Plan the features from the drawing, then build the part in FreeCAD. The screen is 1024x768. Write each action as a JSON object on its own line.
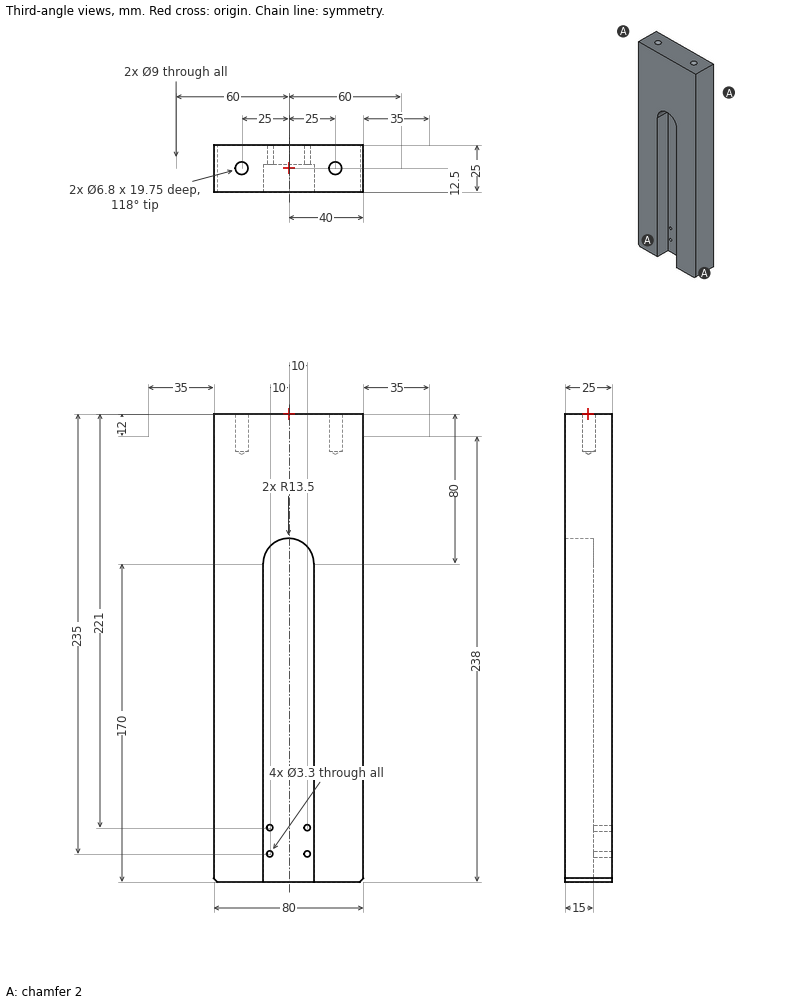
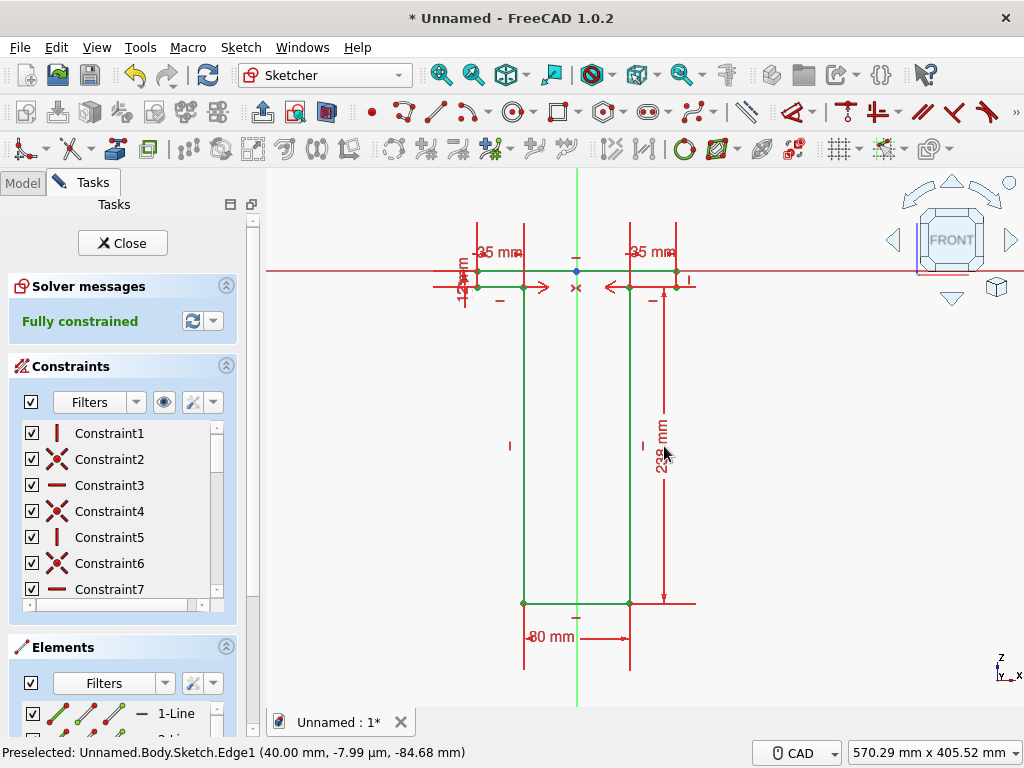
{"action": "left_click", "coordinate": [123, 243]}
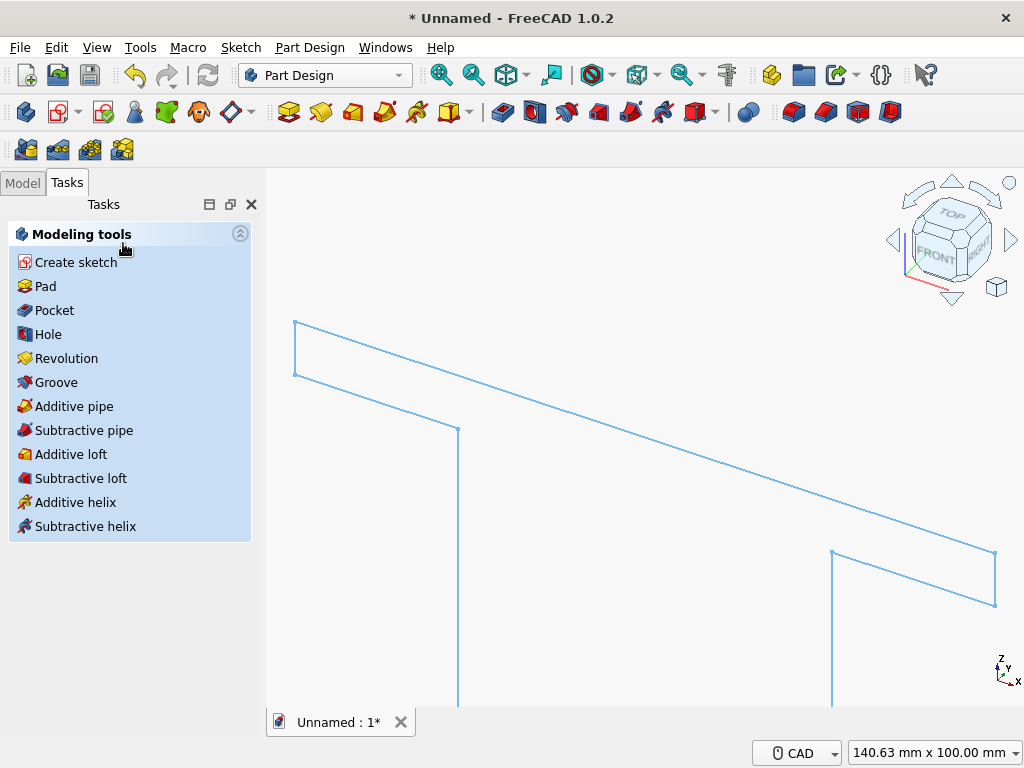
{"action": "left_click", "coordinate": [290, 112]}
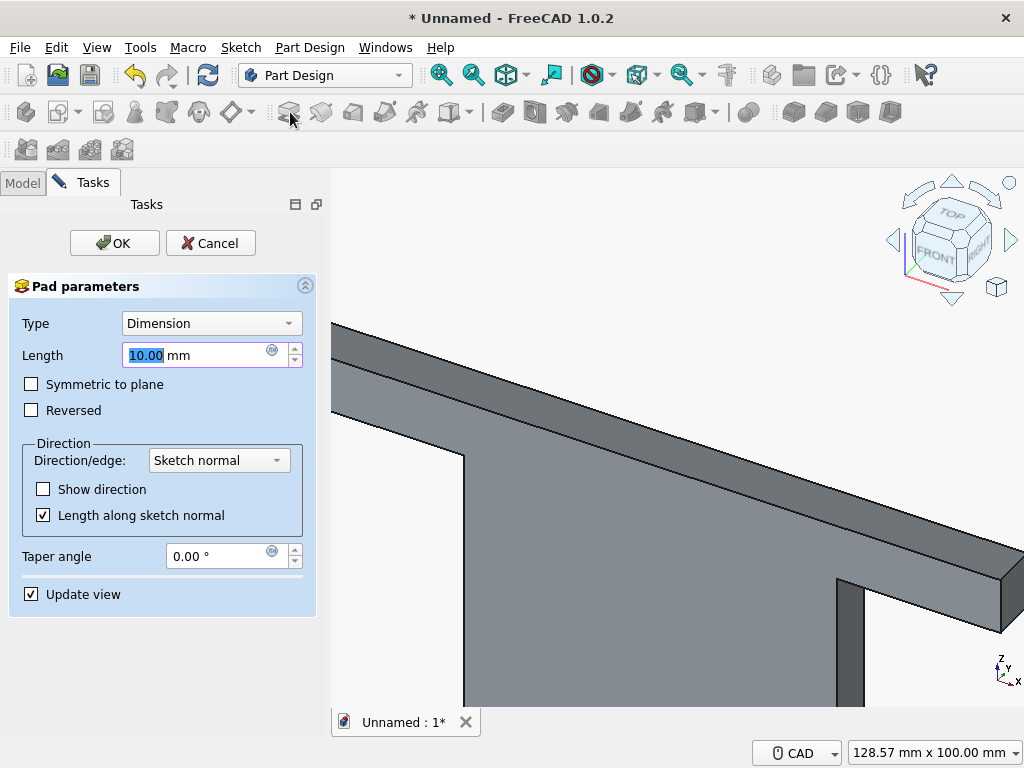
{"action": "type", "text": "25"}
{"action": "key", "text": "Tab"}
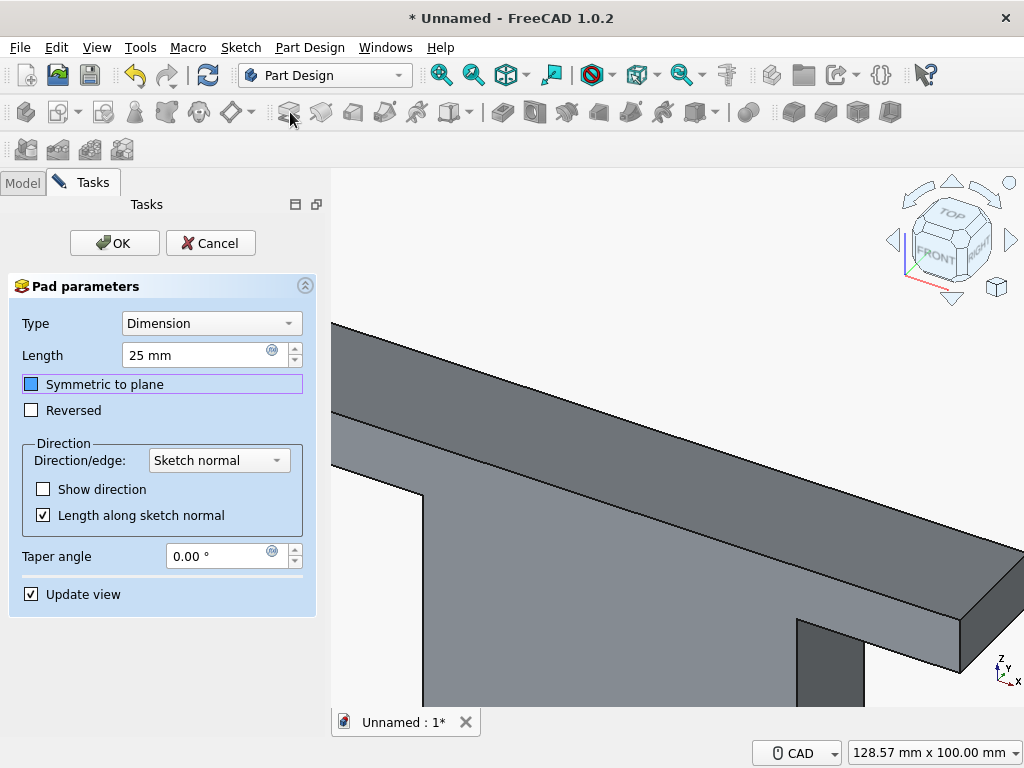
{"action": "left_click", "coordinate": [30, 384]}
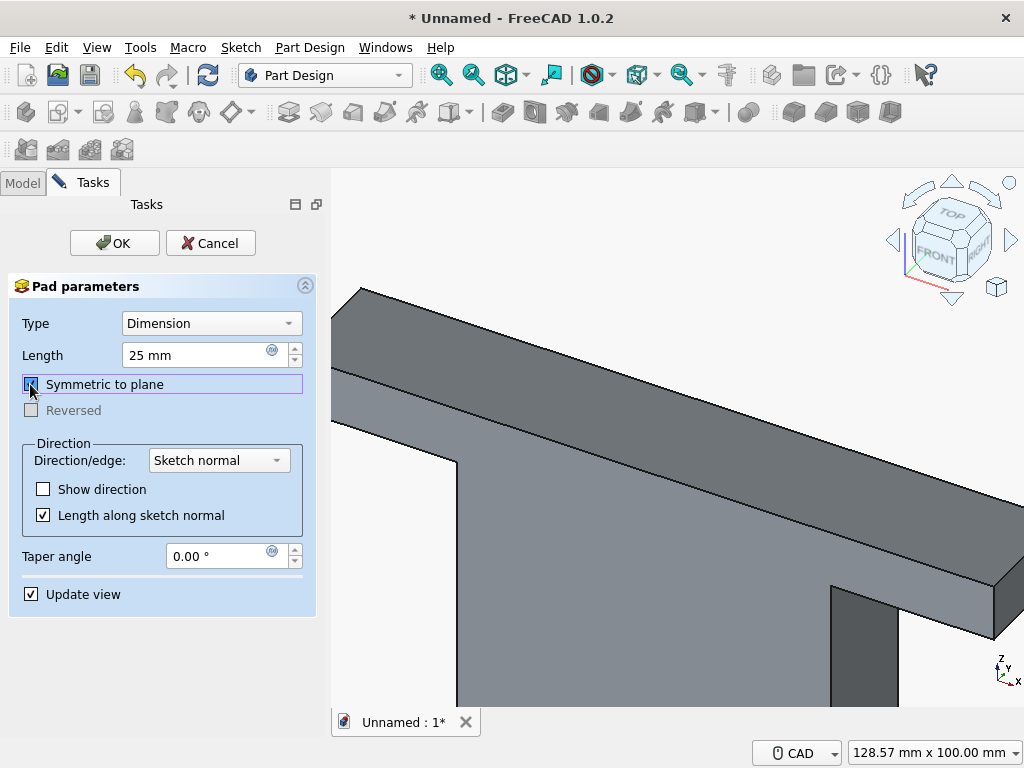
{"action": "left_click", "coordinate": [115, 243]}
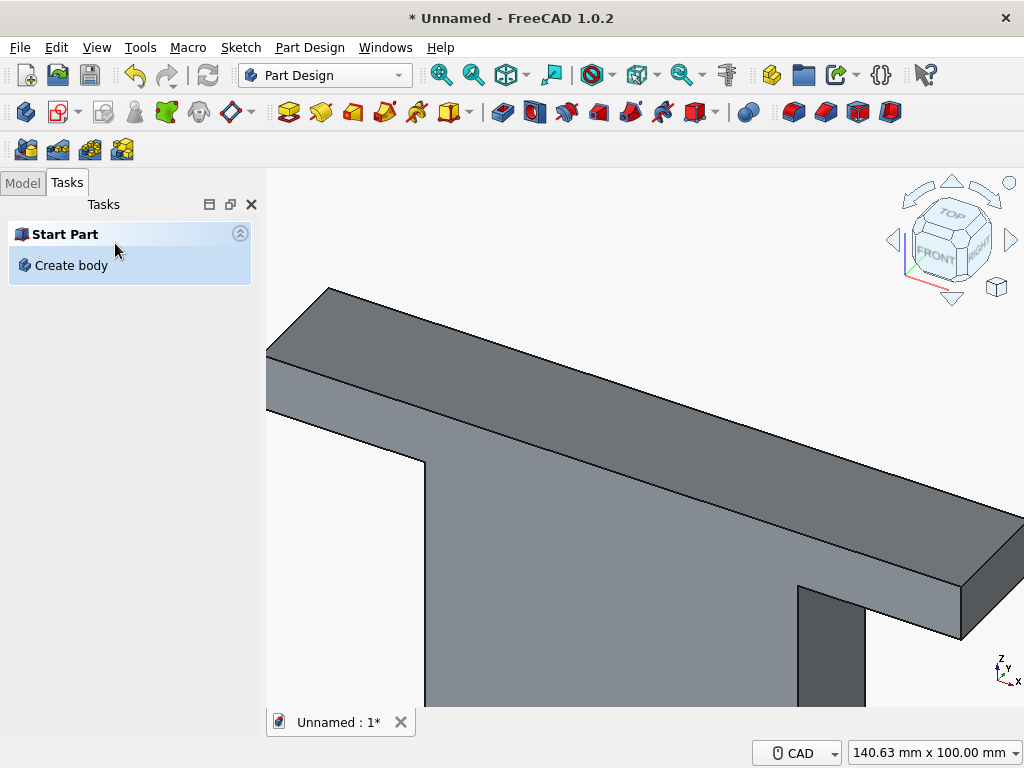
{"action": "key", "text": "v f"}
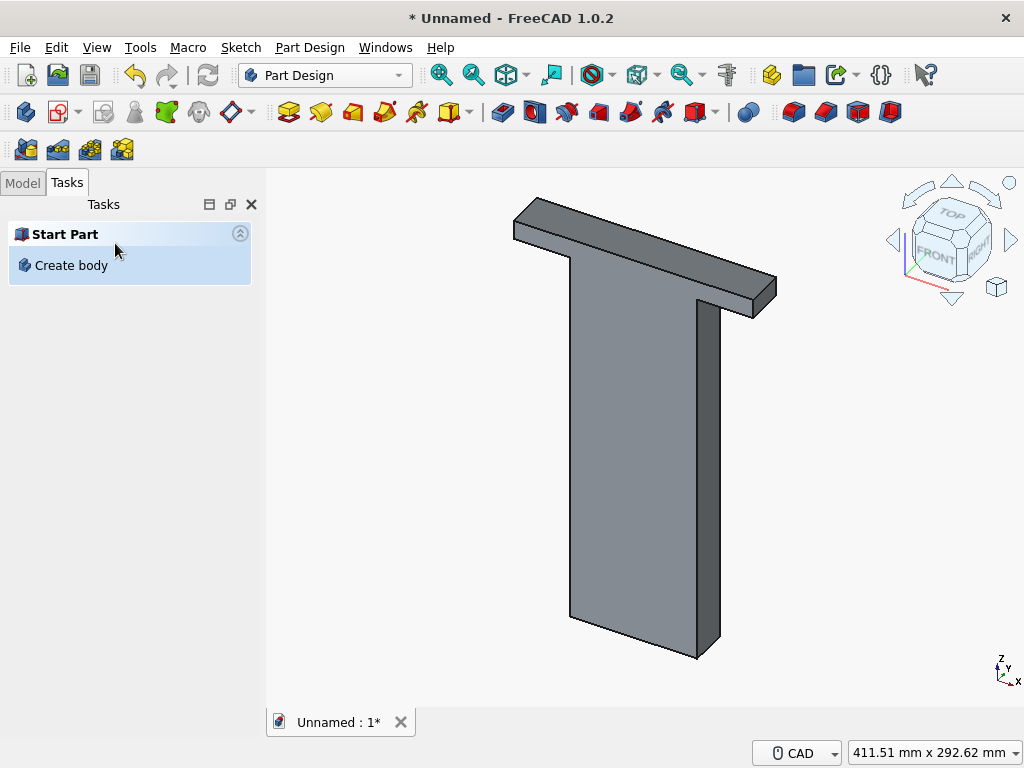
{"action": "key", "text": "0"}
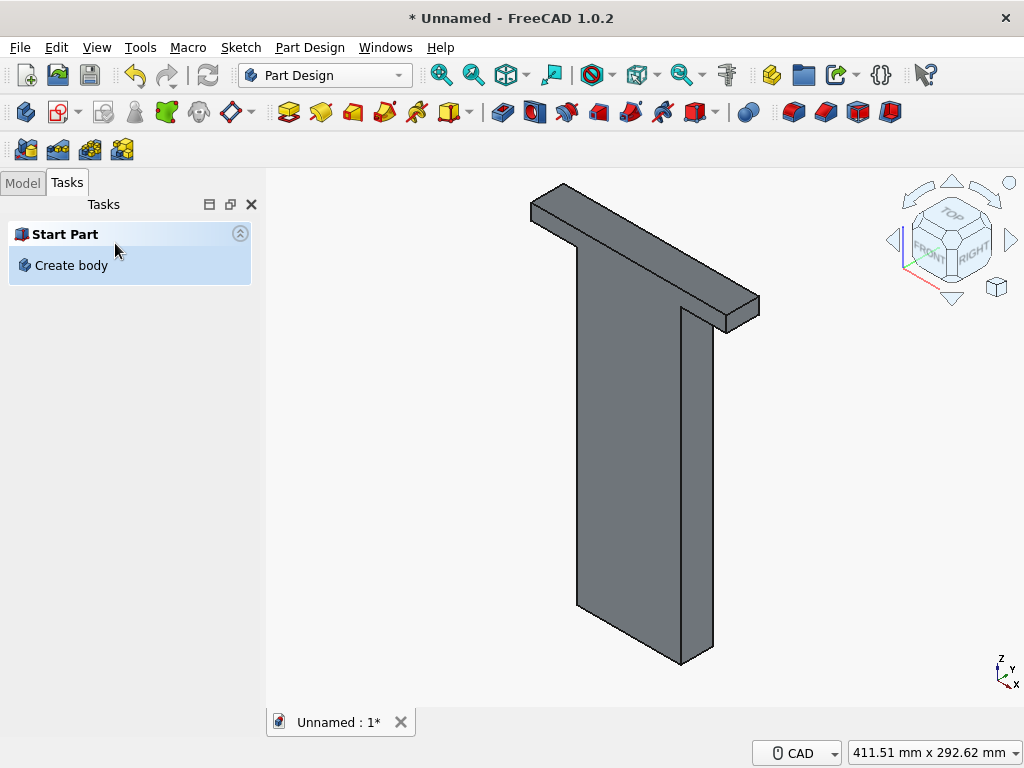
{"action": "key", "text": "2"}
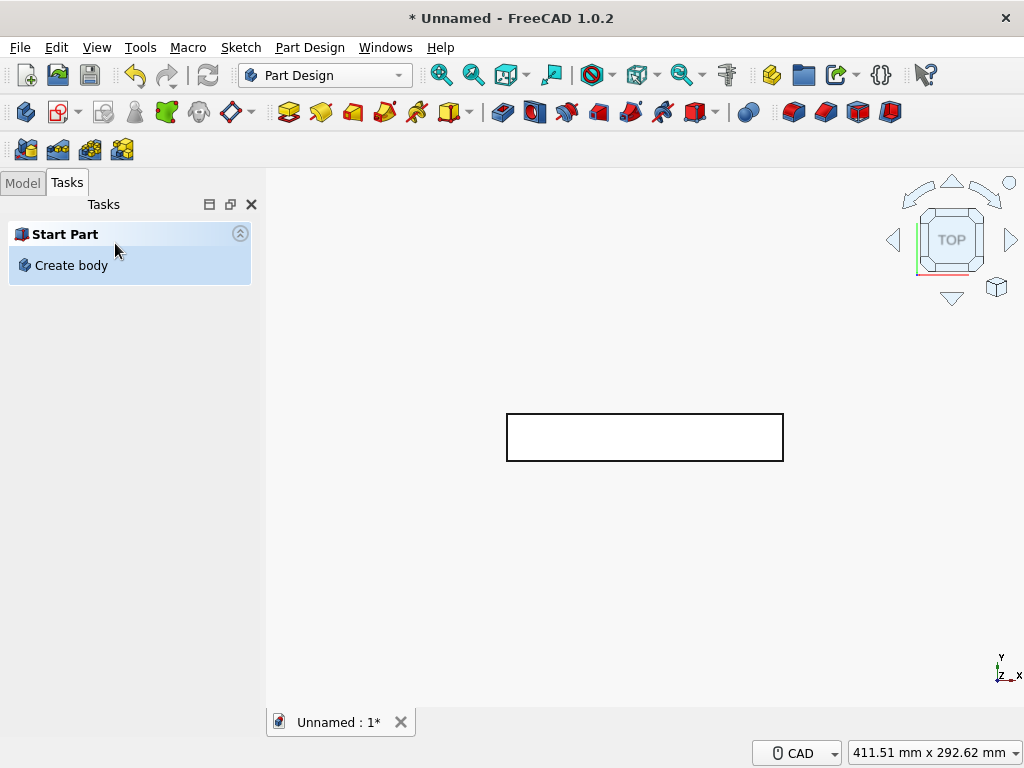
{"action": "left_click", "coordinate": [442, 76]}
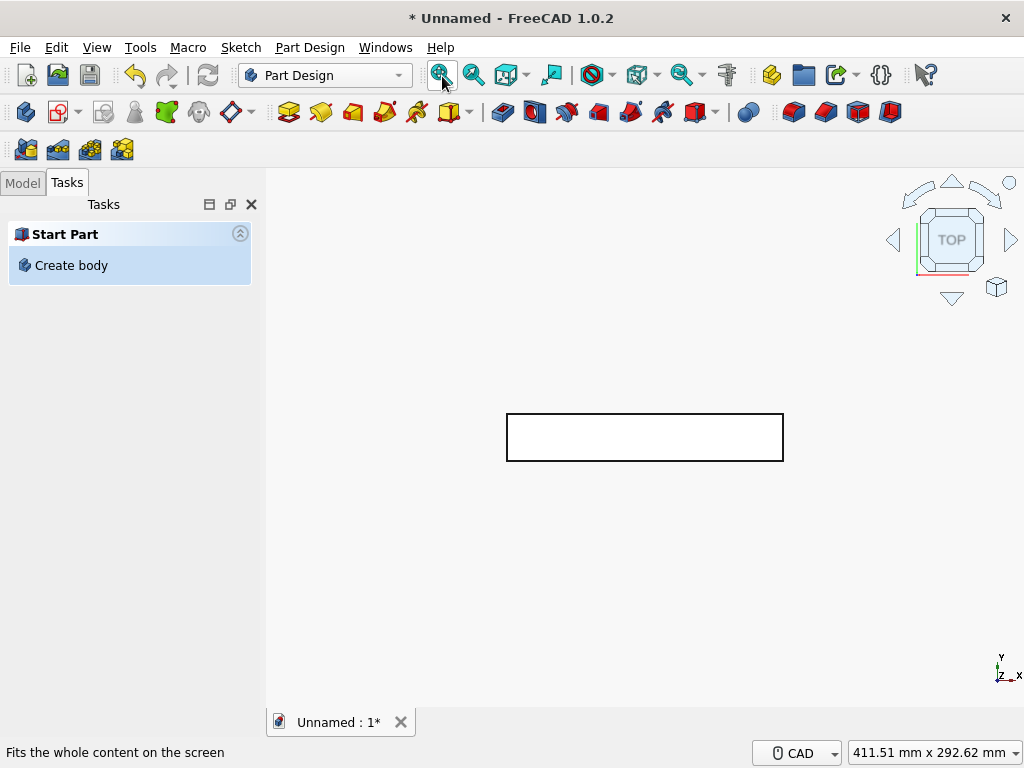
{"action": "key", "text": "1"}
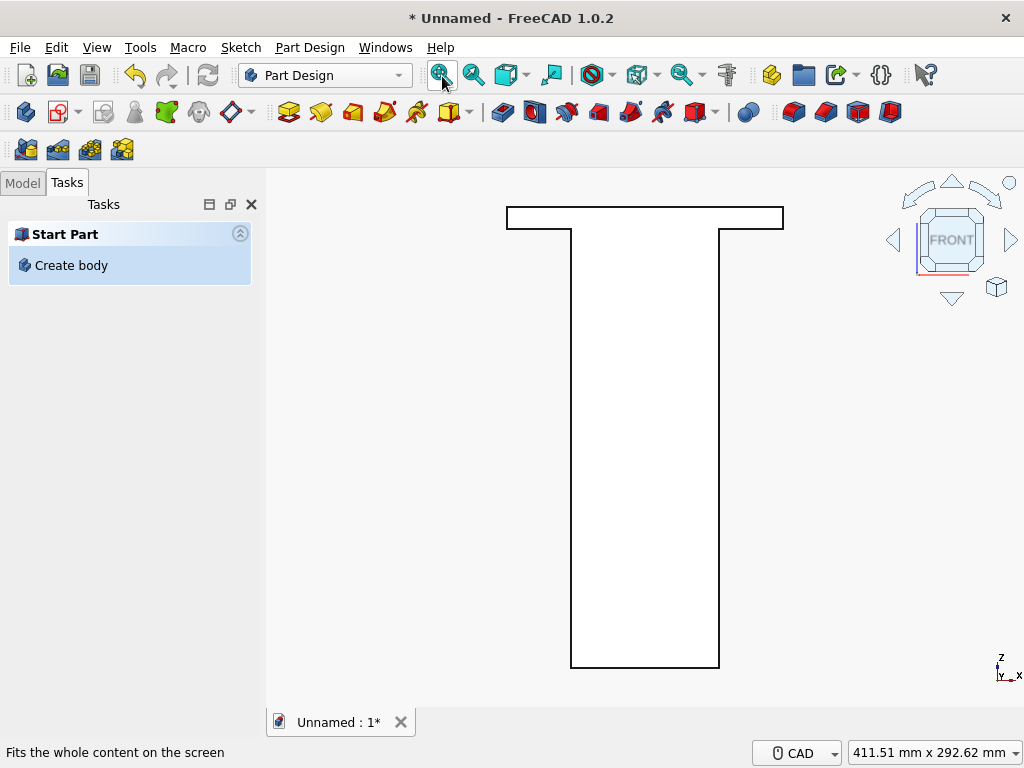
{"action": "key", "text": "3"}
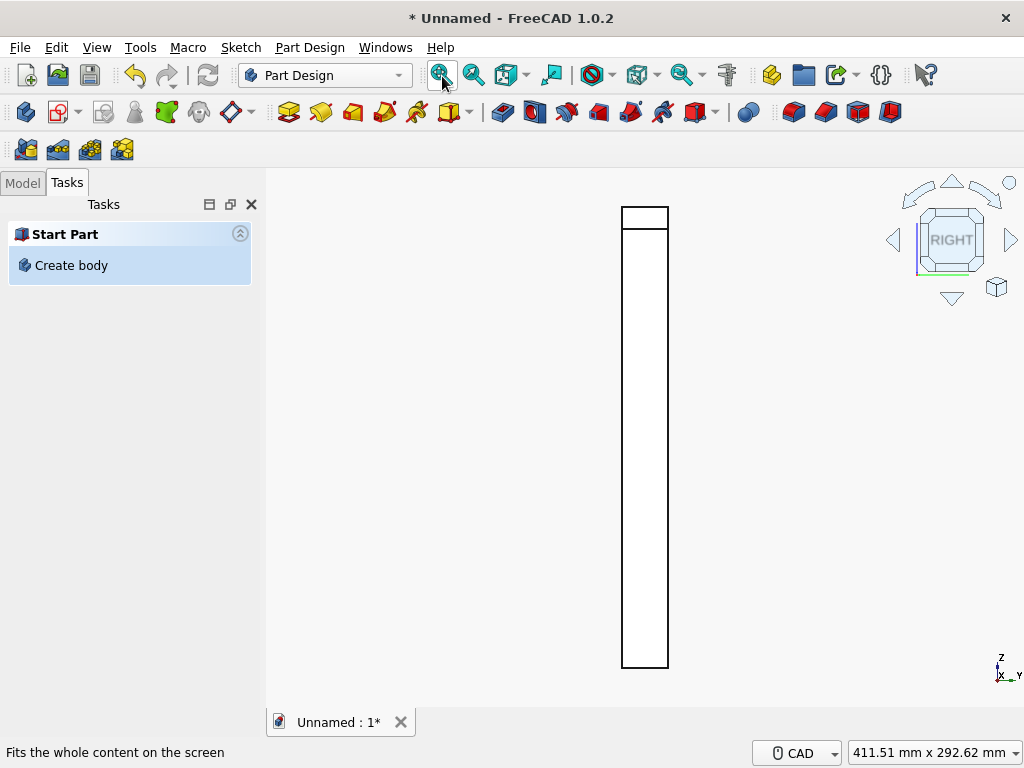
{"action": "left_click", "coordinate": [645, 667]}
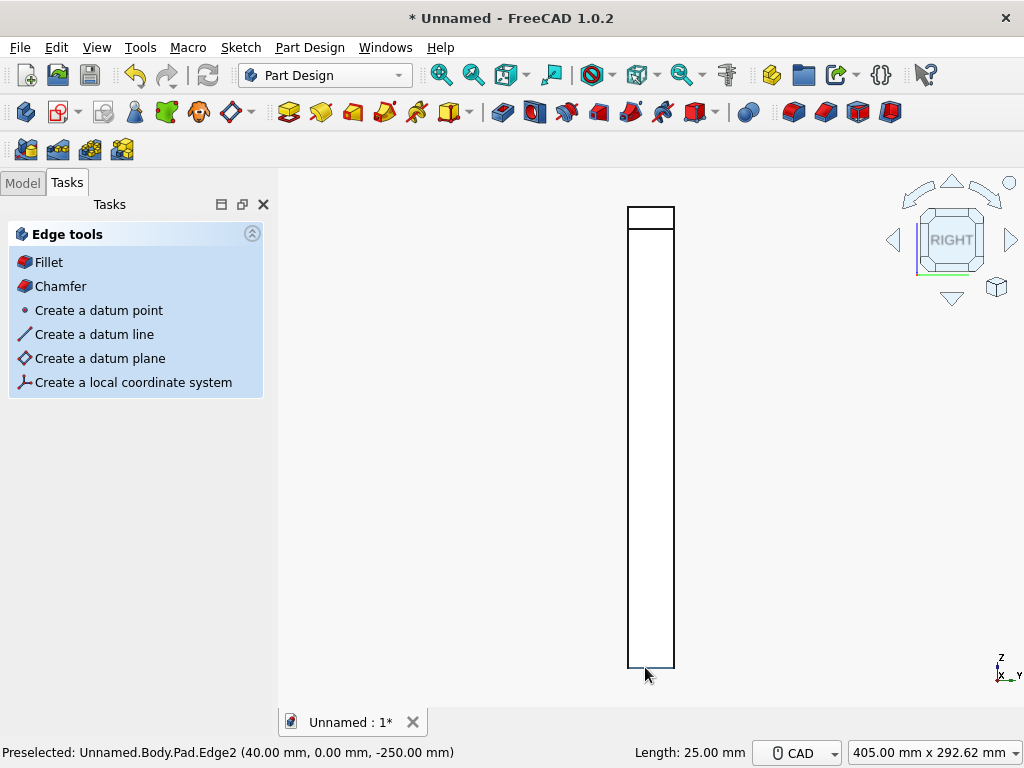
{"action": "left_click", "coordinate": [651, 228], "text": "ctrl"}